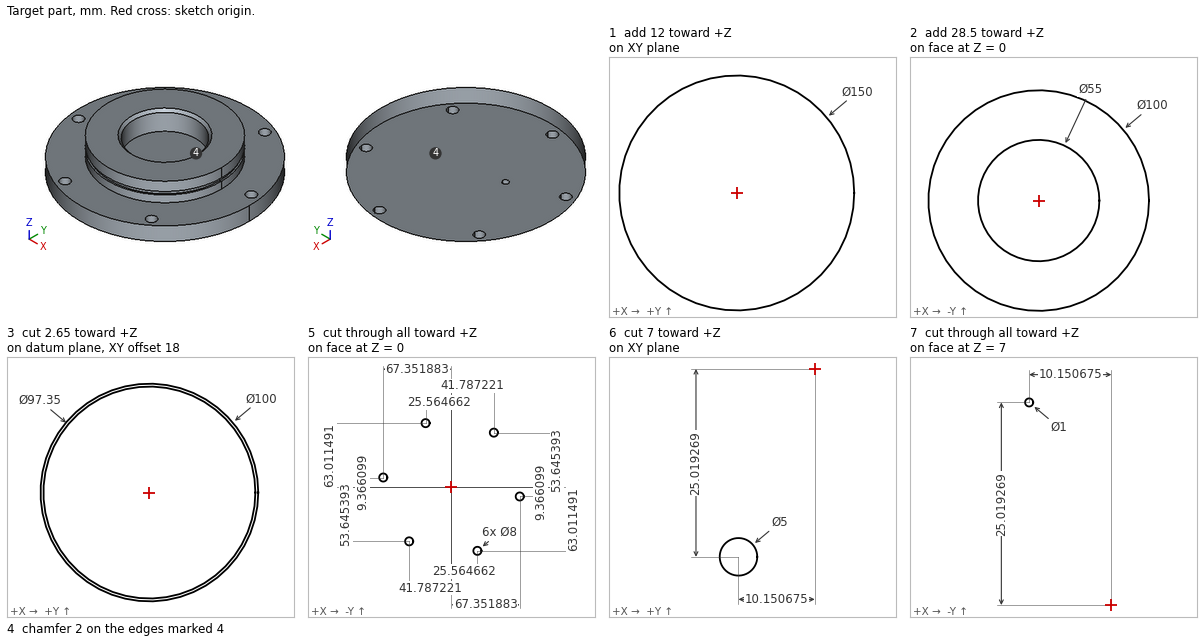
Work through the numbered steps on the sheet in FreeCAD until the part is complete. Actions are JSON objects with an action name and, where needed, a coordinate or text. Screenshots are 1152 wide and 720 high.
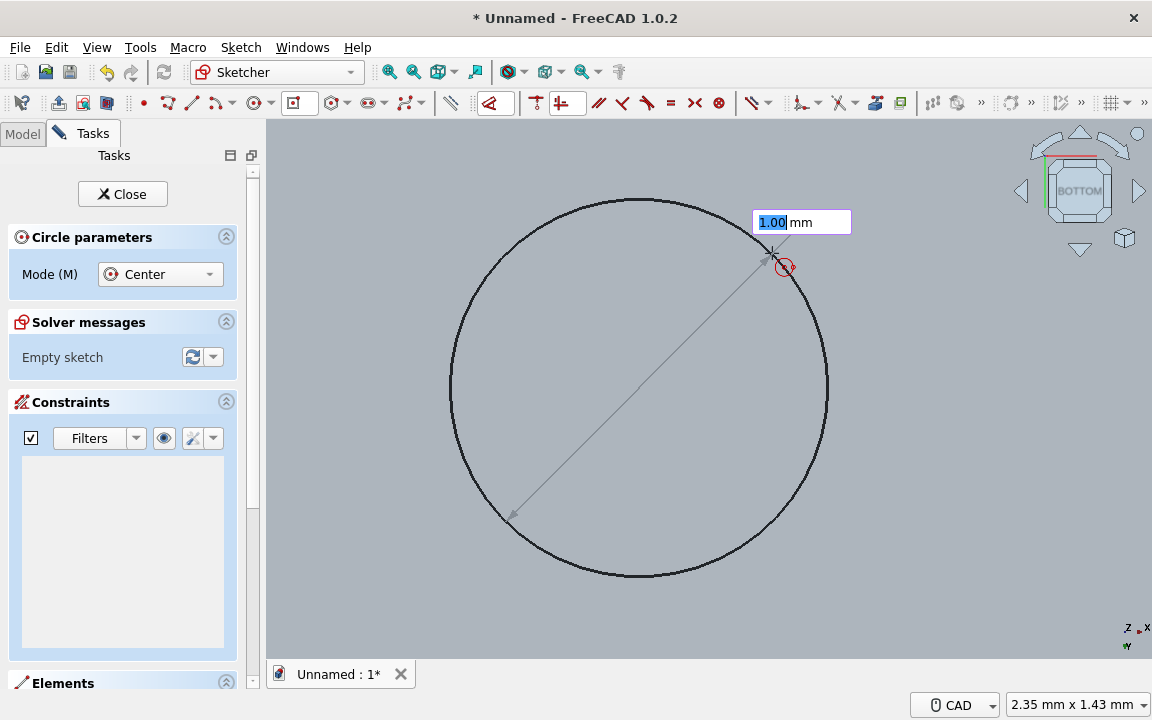
{"action": "type", "text": "1"}
{"action": "key", "text": "Return"}
{"action": "key", "text": "Escape"}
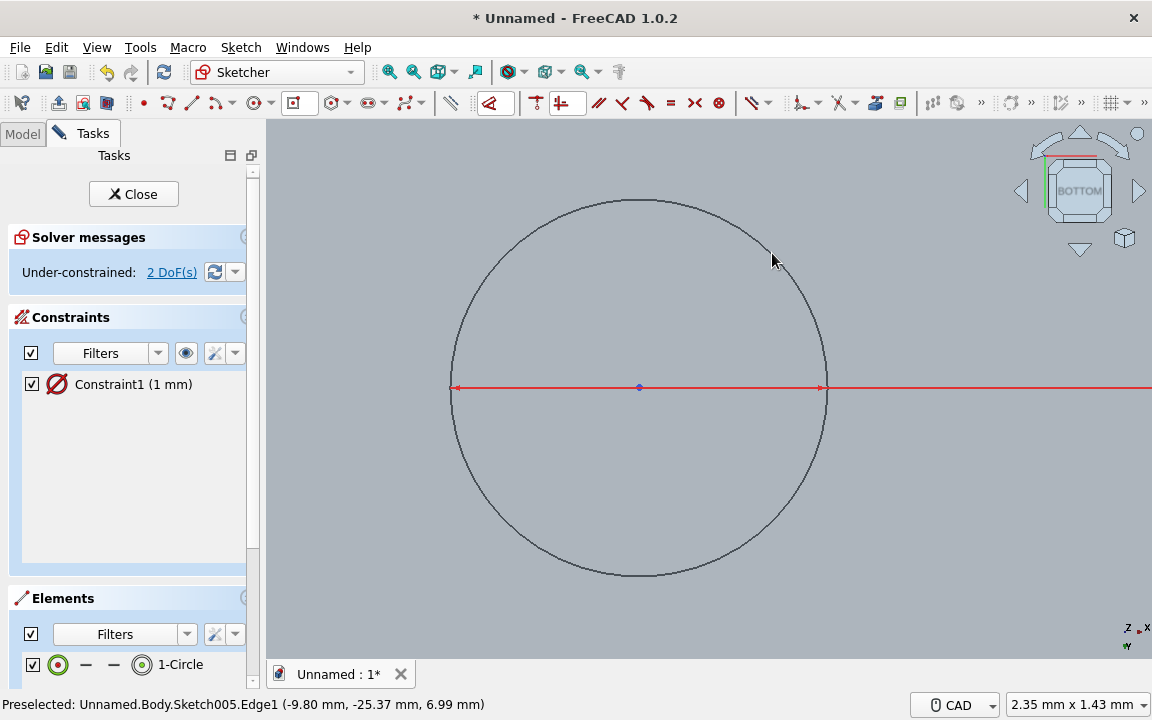
{"action": "left_click", "coordinate": [639, 388]}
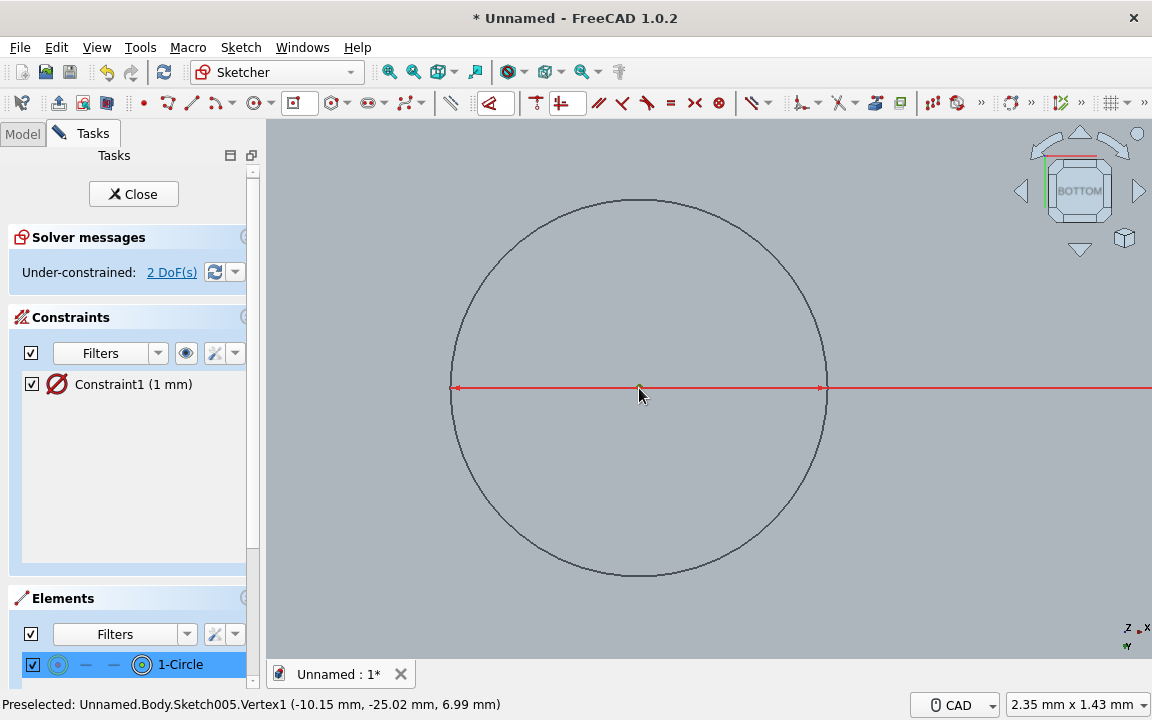
{"action": "key", "text": "l"}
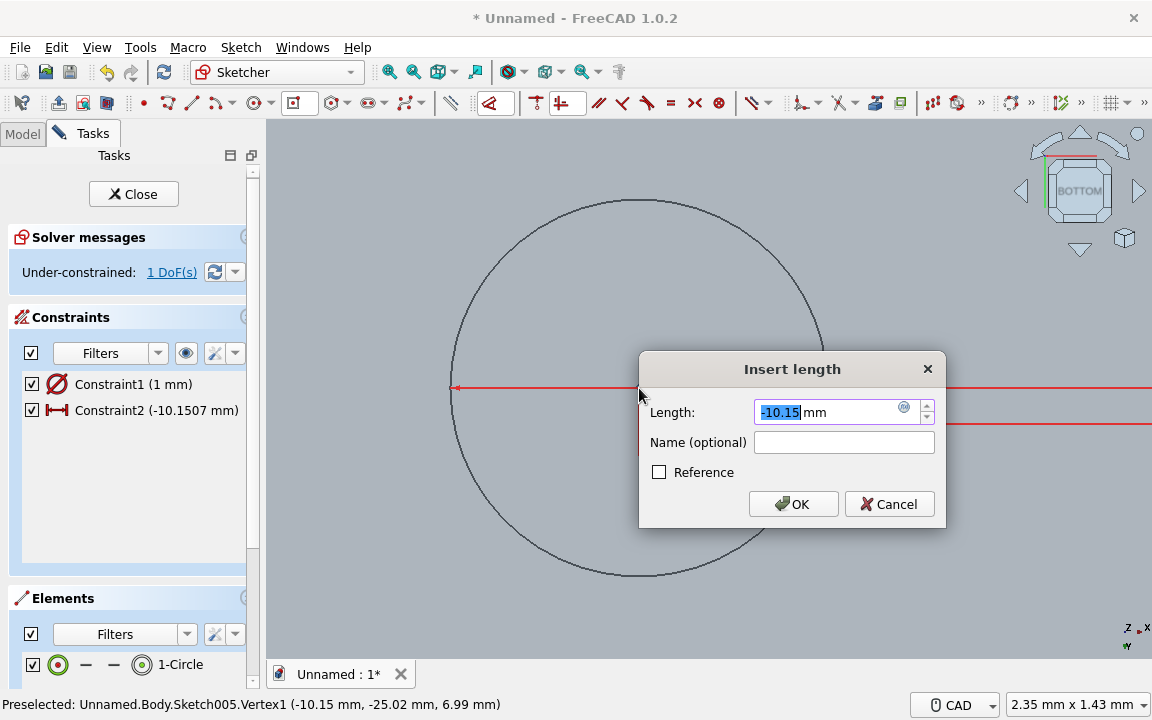
{"action": "type", "text": "-10.150675"}
{"action": "key", "text": "Return"}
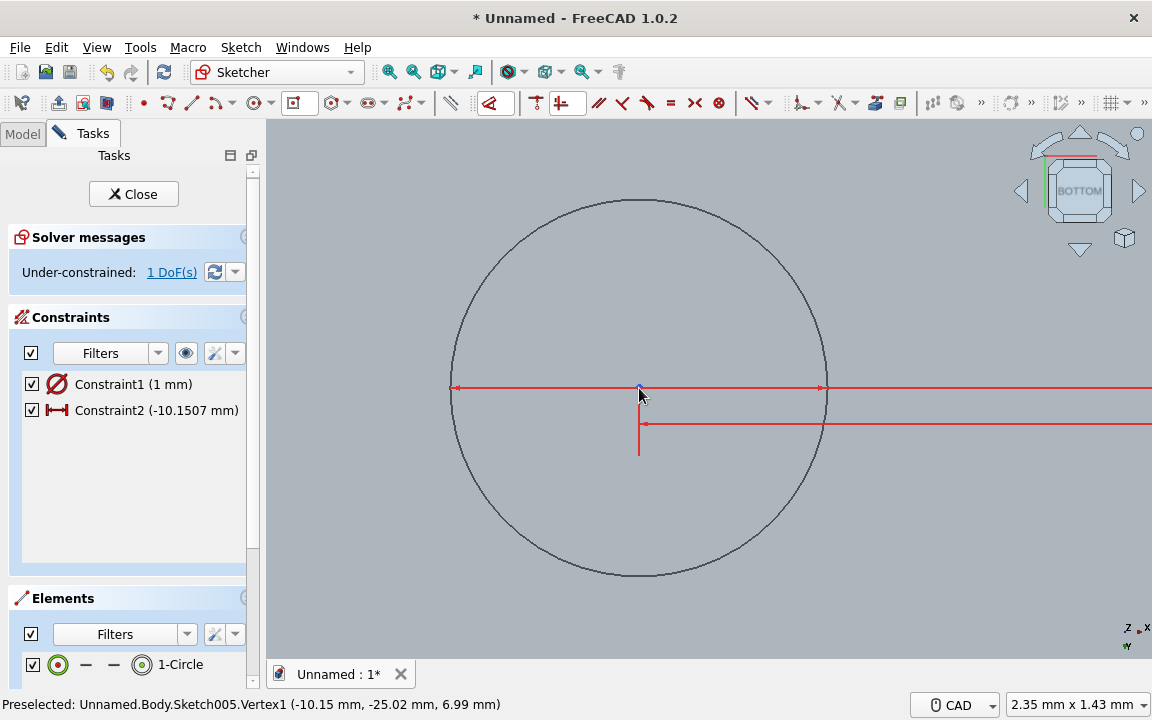
{"action": "left_click", "coordinate": [639, 388]}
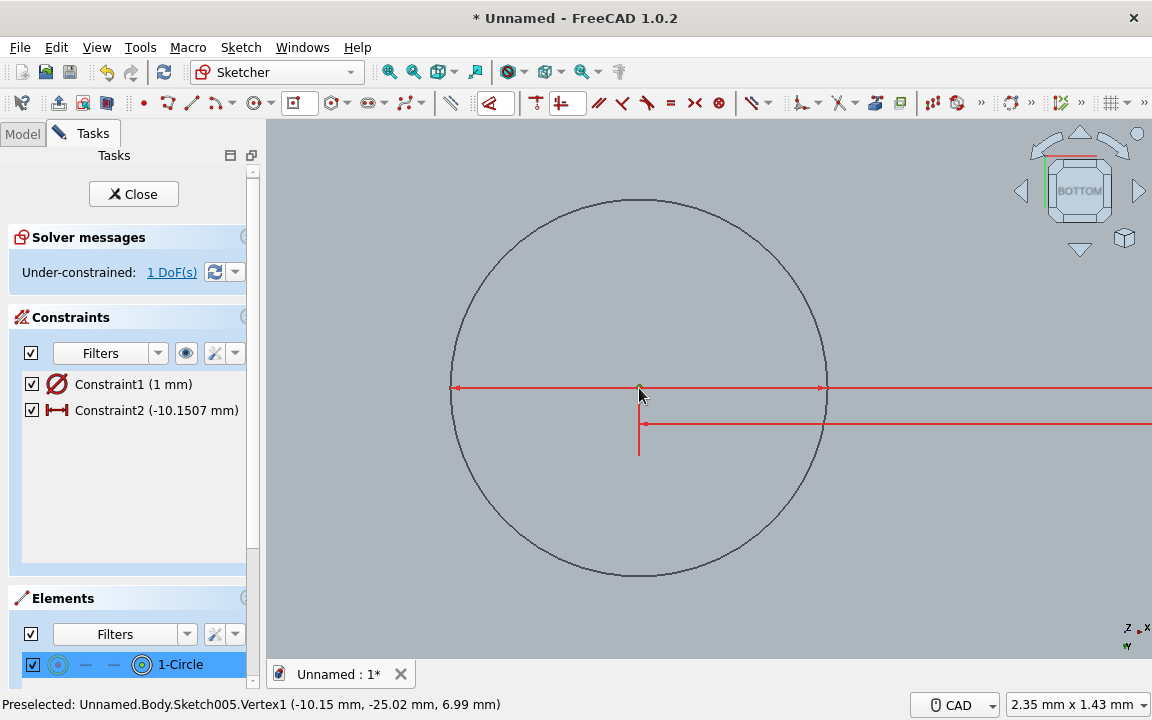
{"action": "key", "text": "i"}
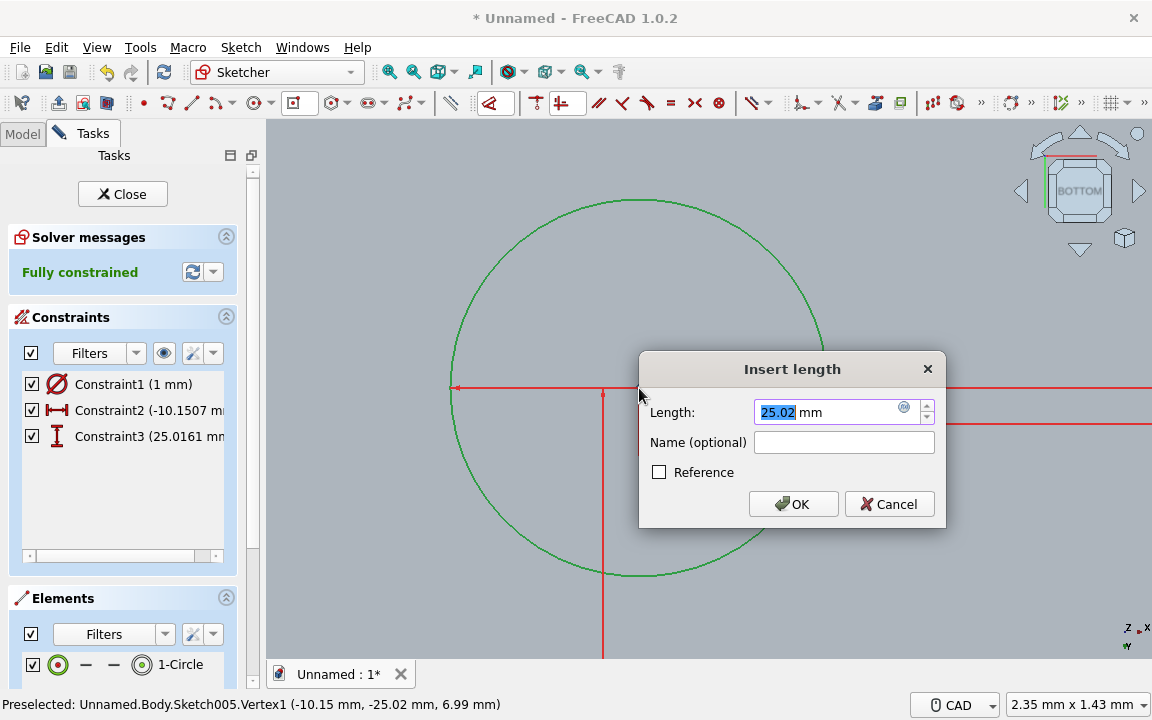
{"action": "type", "text": "25.019269"}
{"action": "key", "text": "Return"}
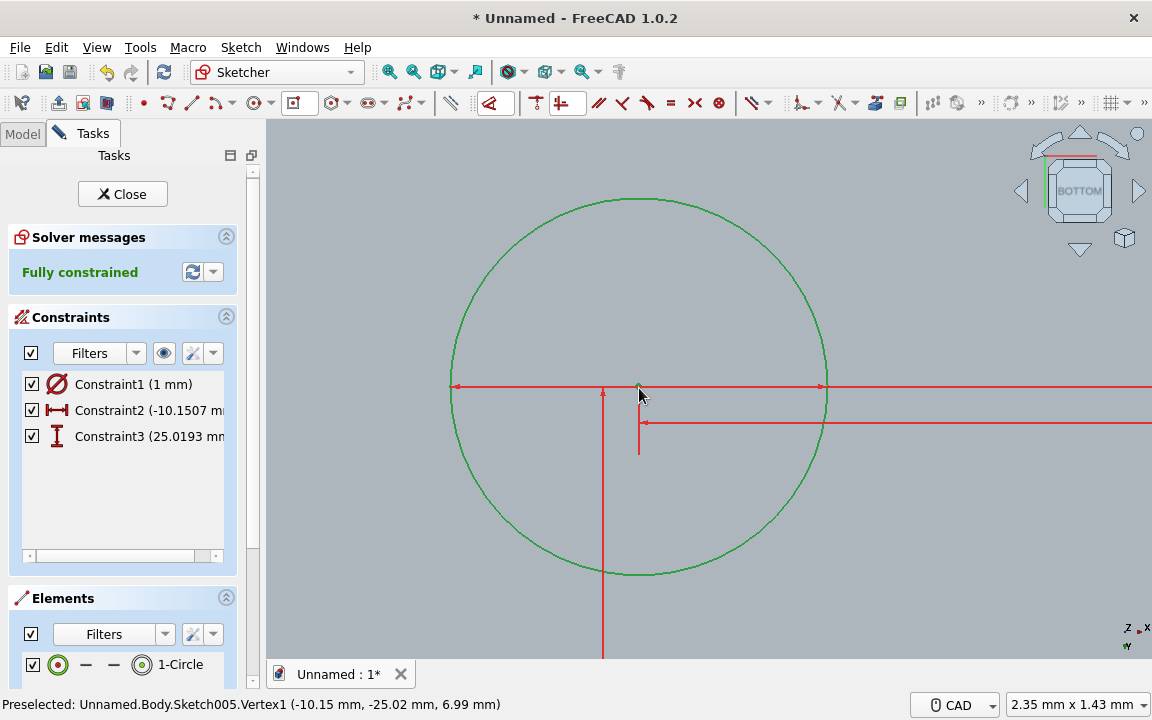
{"action": "left_click", "coordinate": [123, 194]}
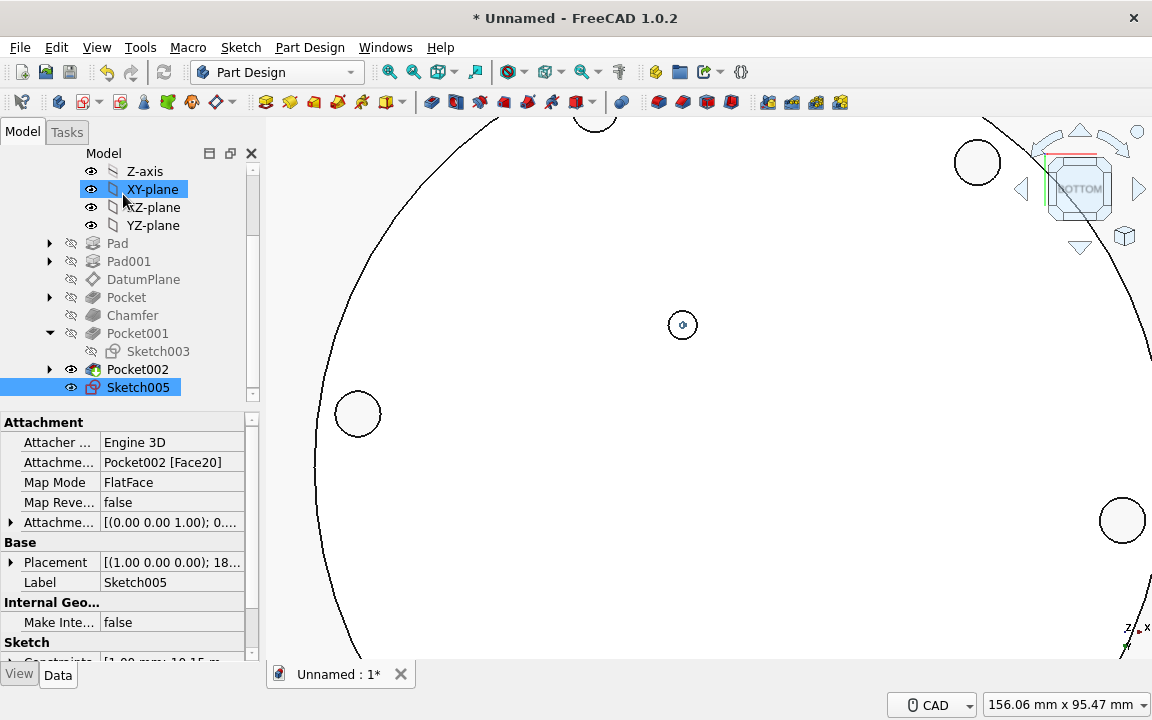
{"action": "left_click", "coordinate": [432, 102]}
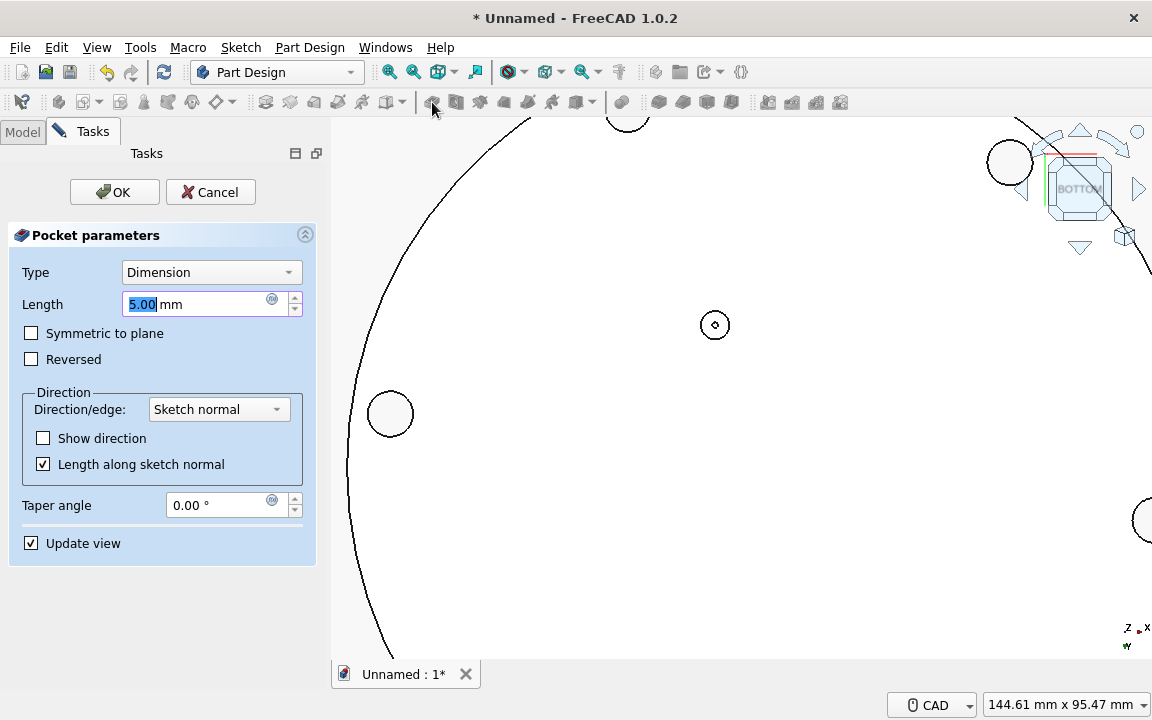
{"action": "left_click", "coordinate": [212, 272]}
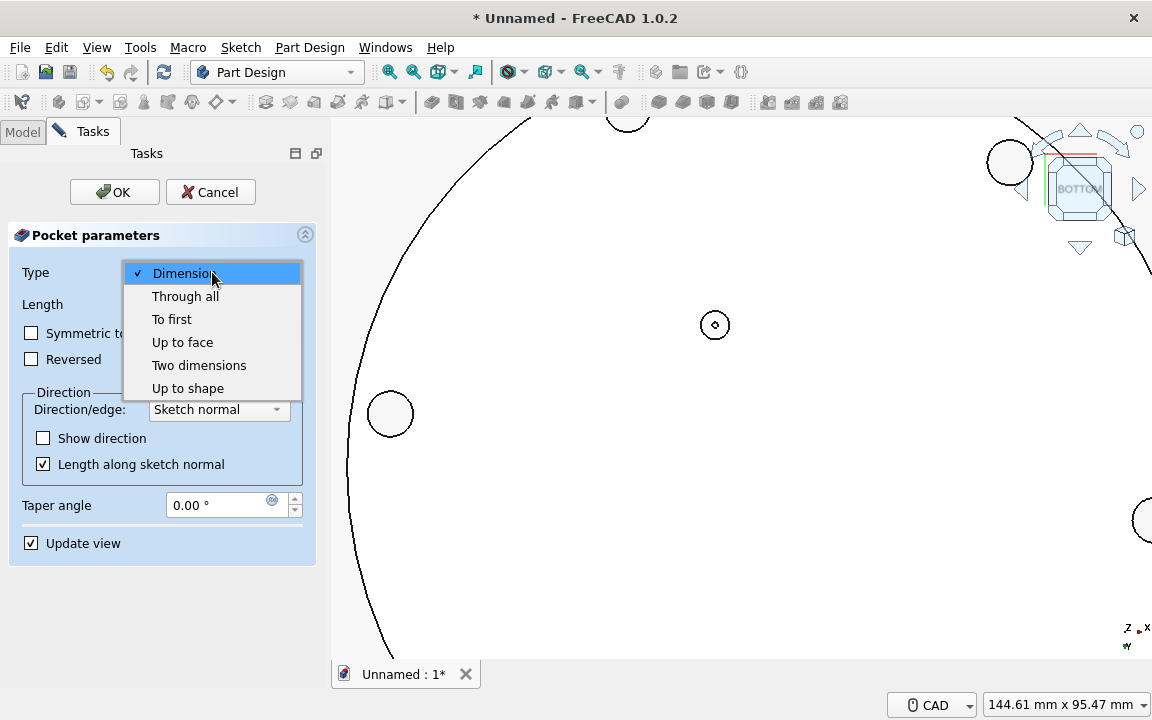
{"action": "left_click", "coordinate": [212, 296]}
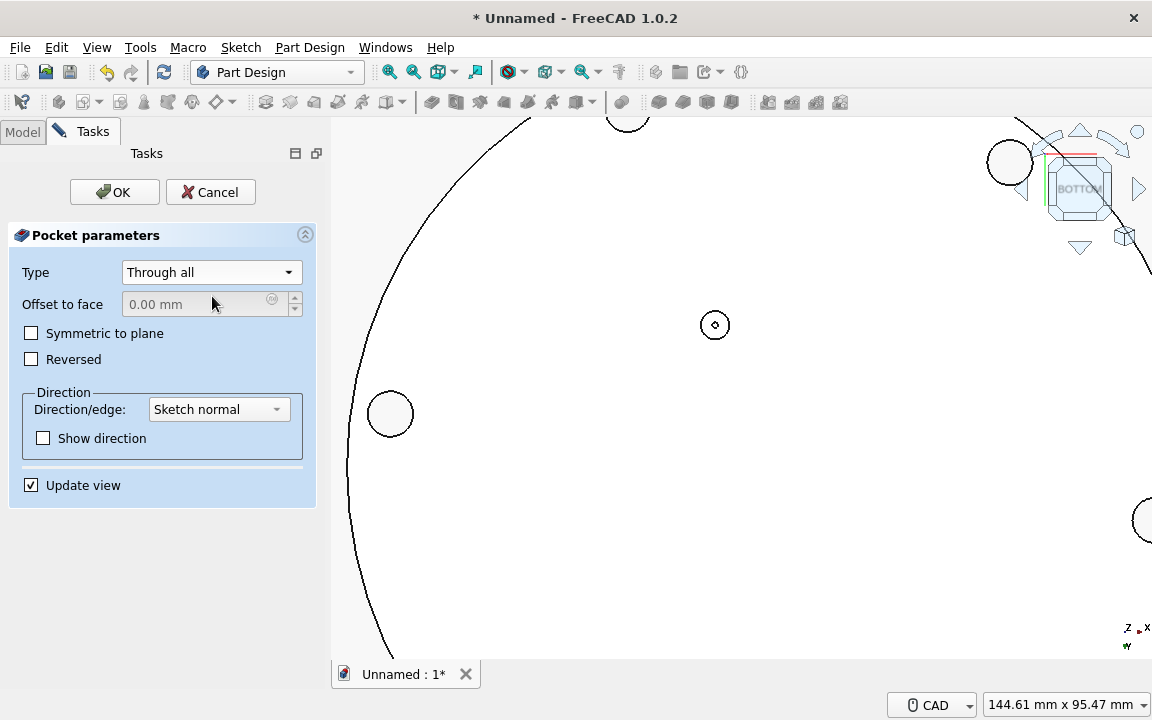
{"action": "left_click", "coordinate": [115, 192]}